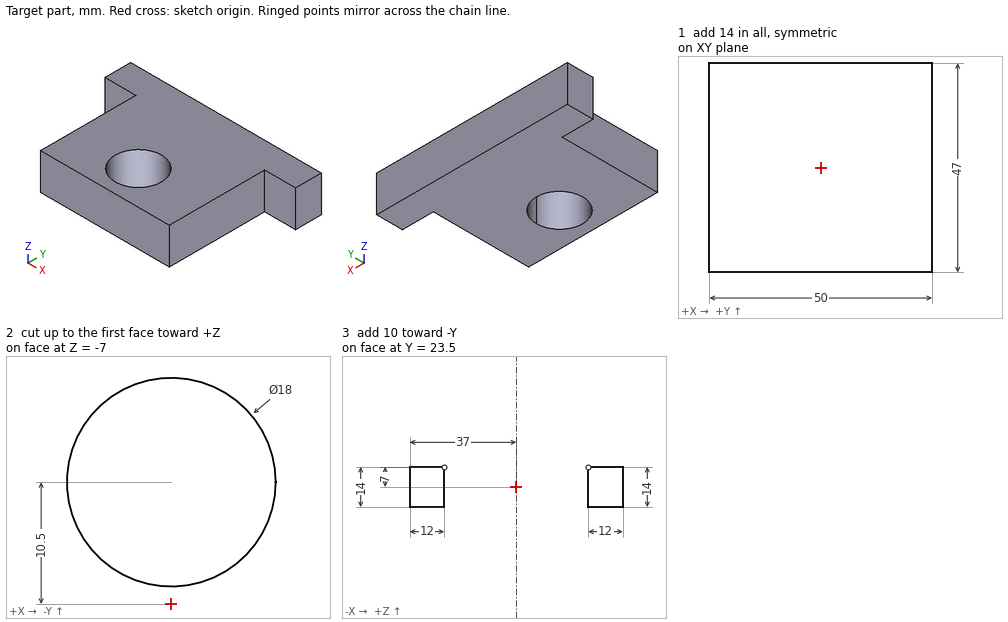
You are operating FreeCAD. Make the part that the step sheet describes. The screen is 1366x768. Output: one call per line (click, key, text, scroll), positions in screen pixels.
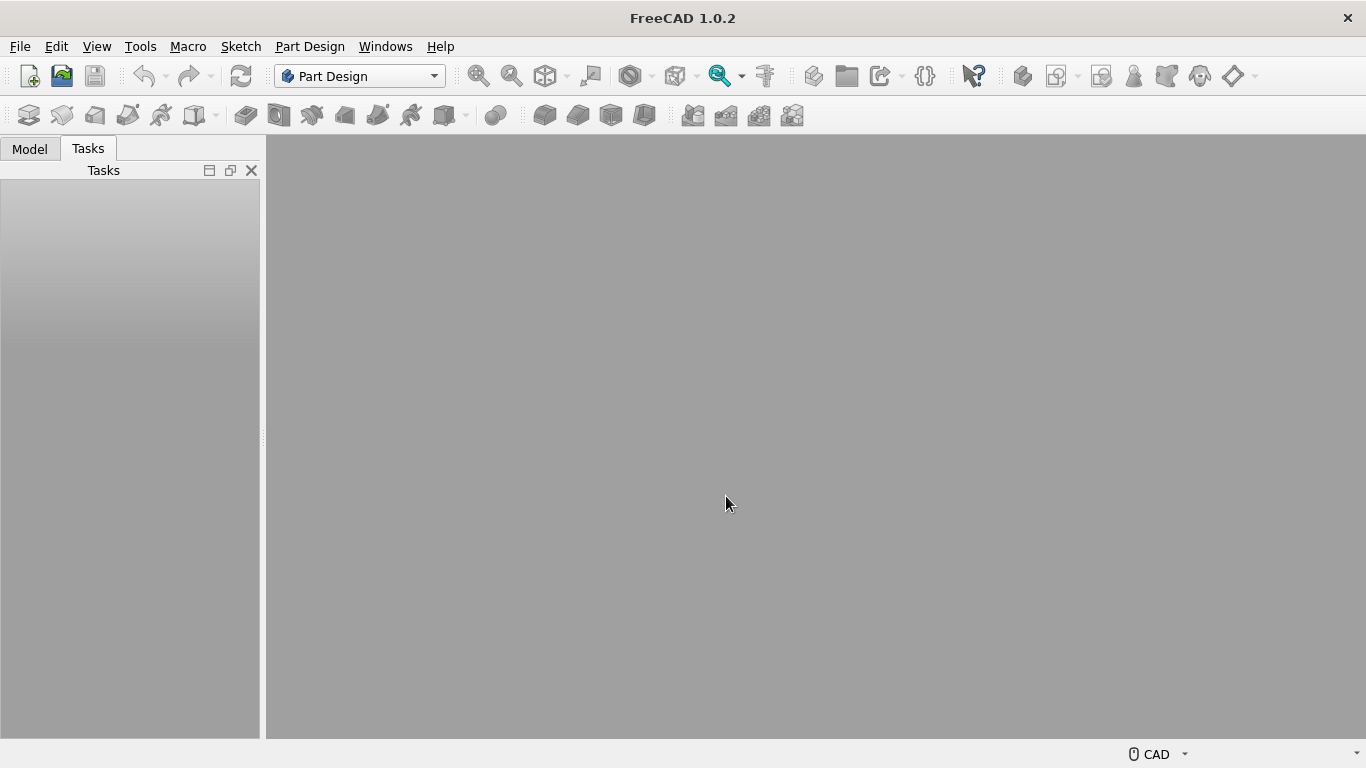
click(29, 76)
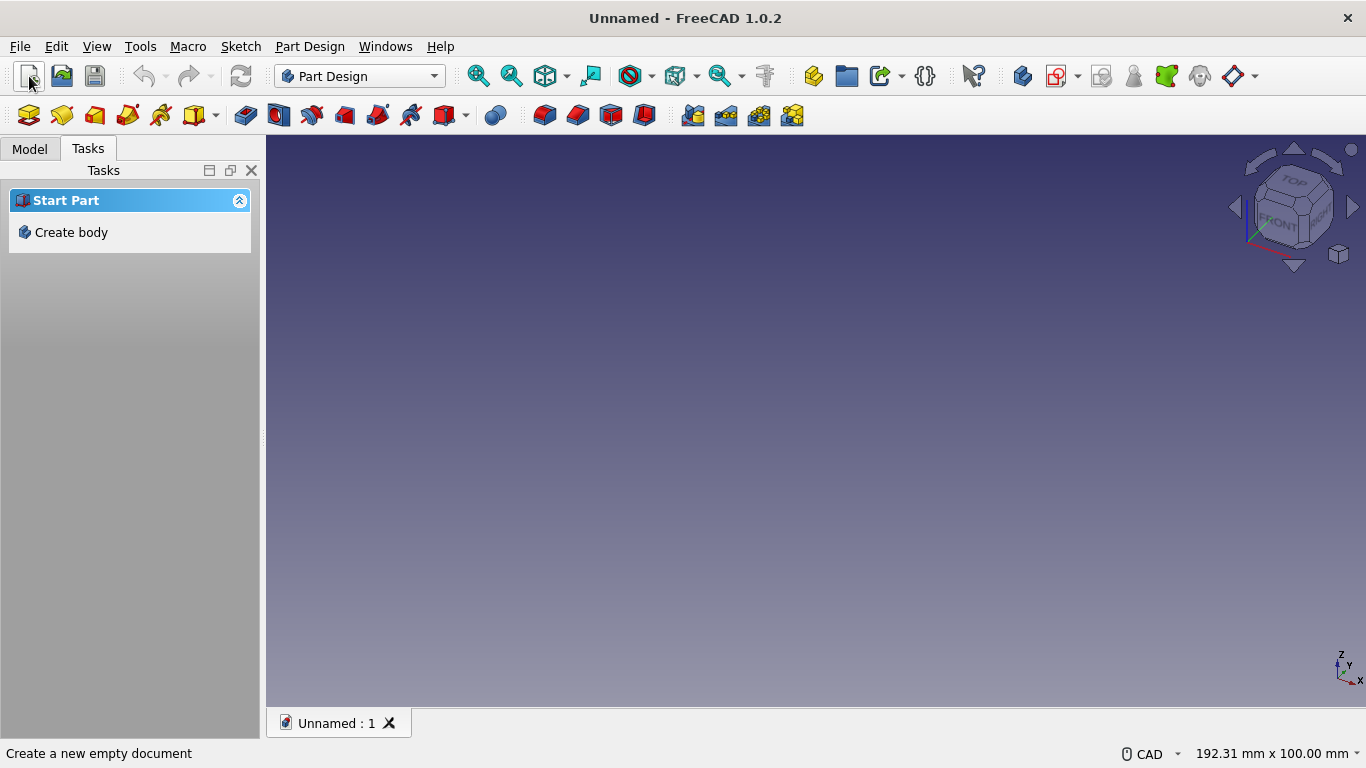
click(1056, 76)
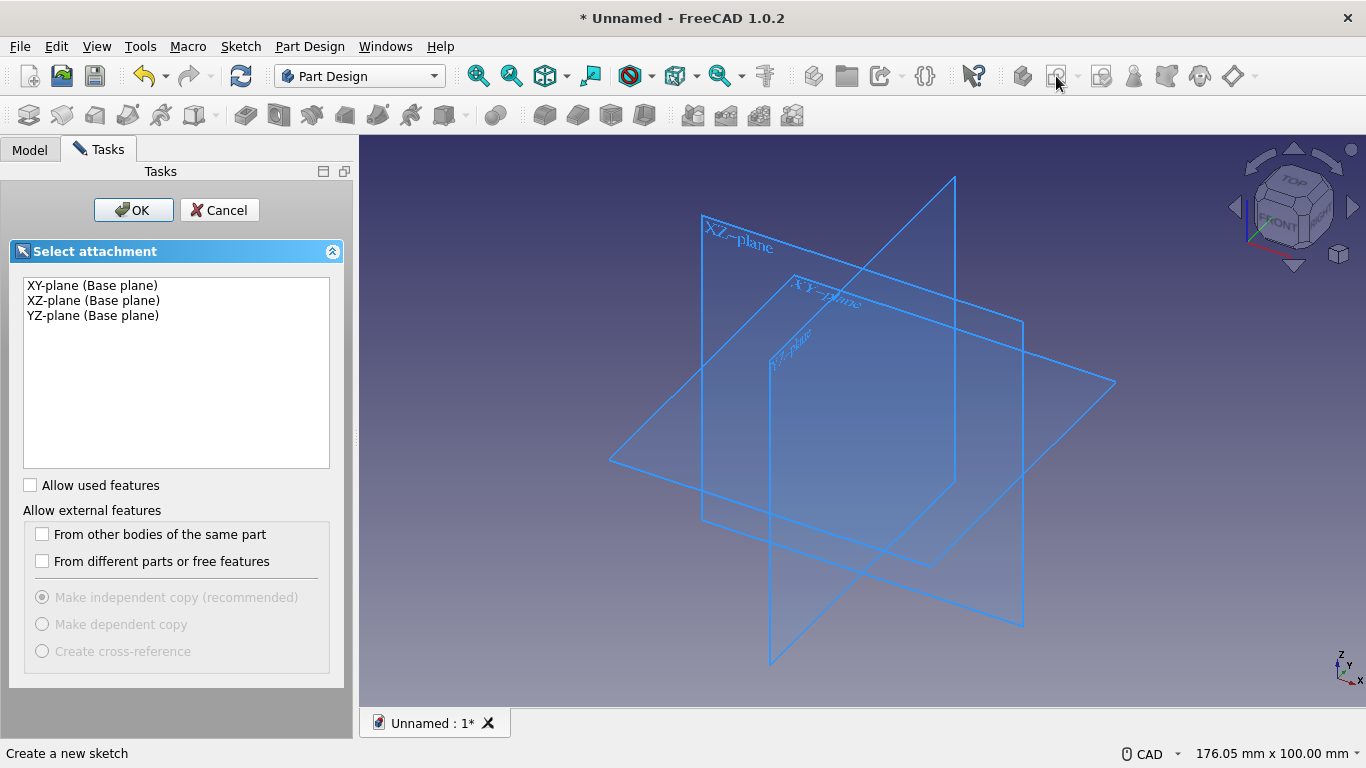
click(84, 286)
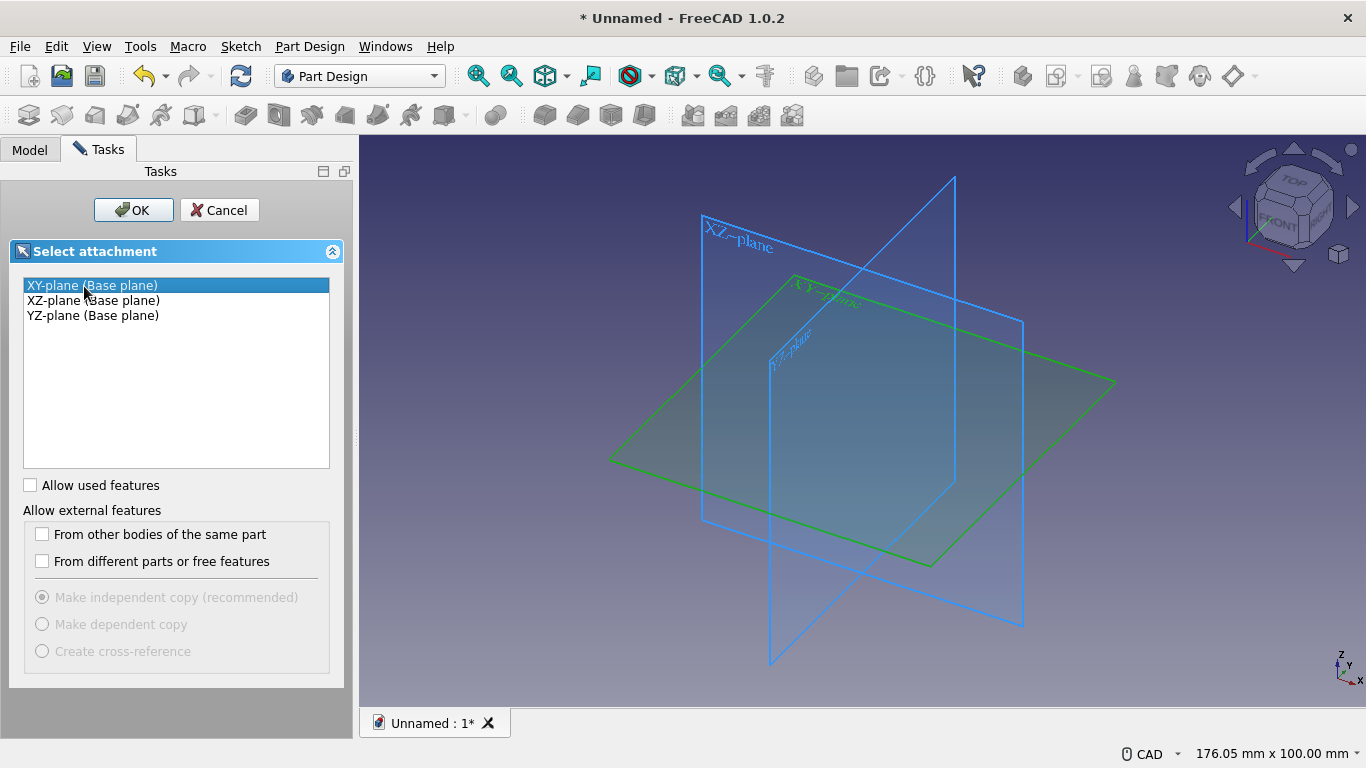
click(134, 210)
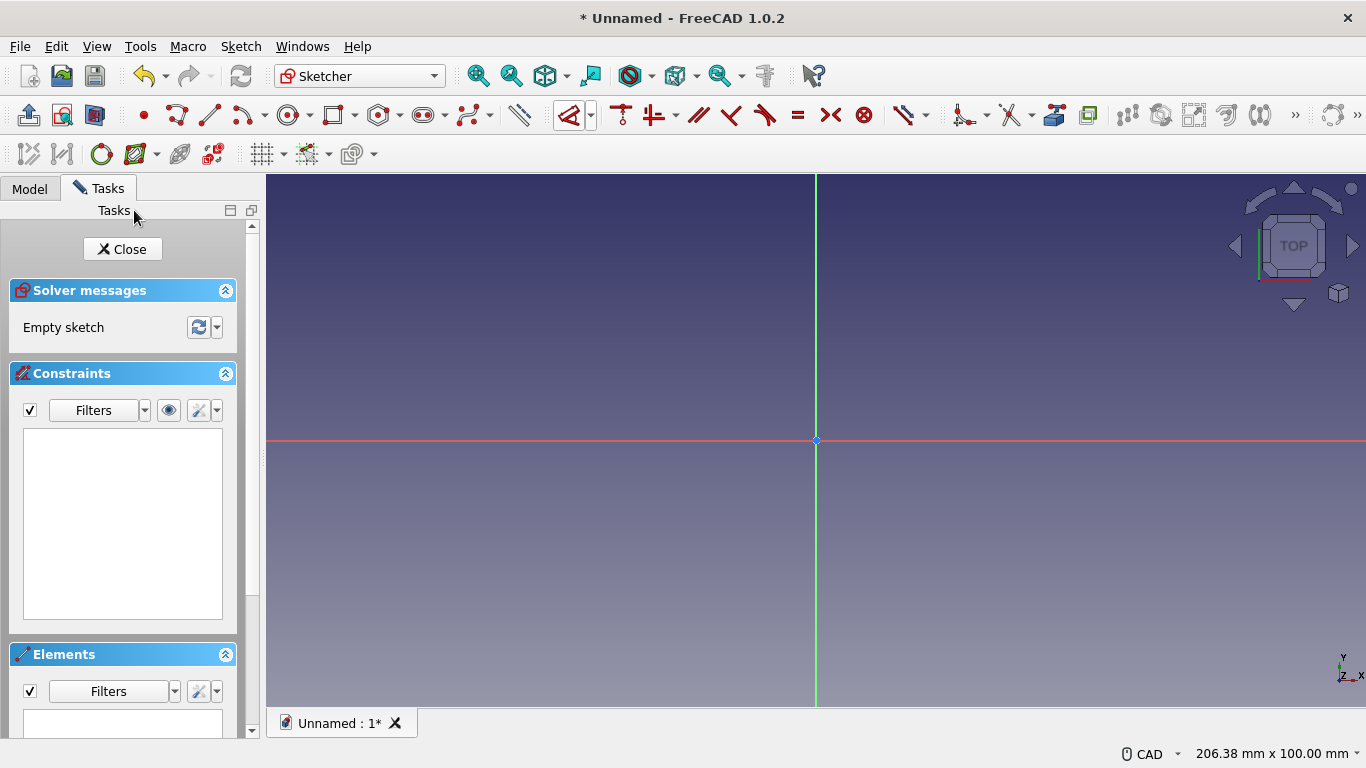
click(354, 116)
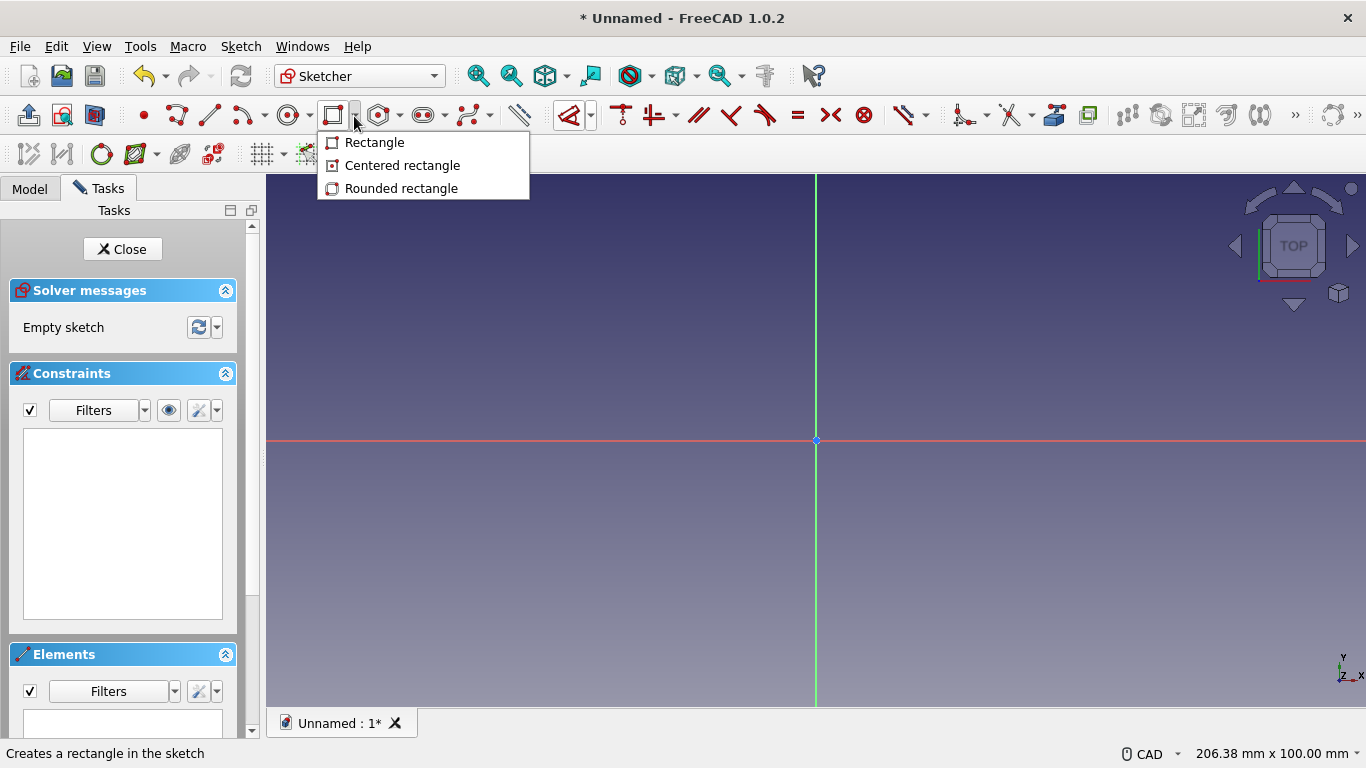
click(424, 166)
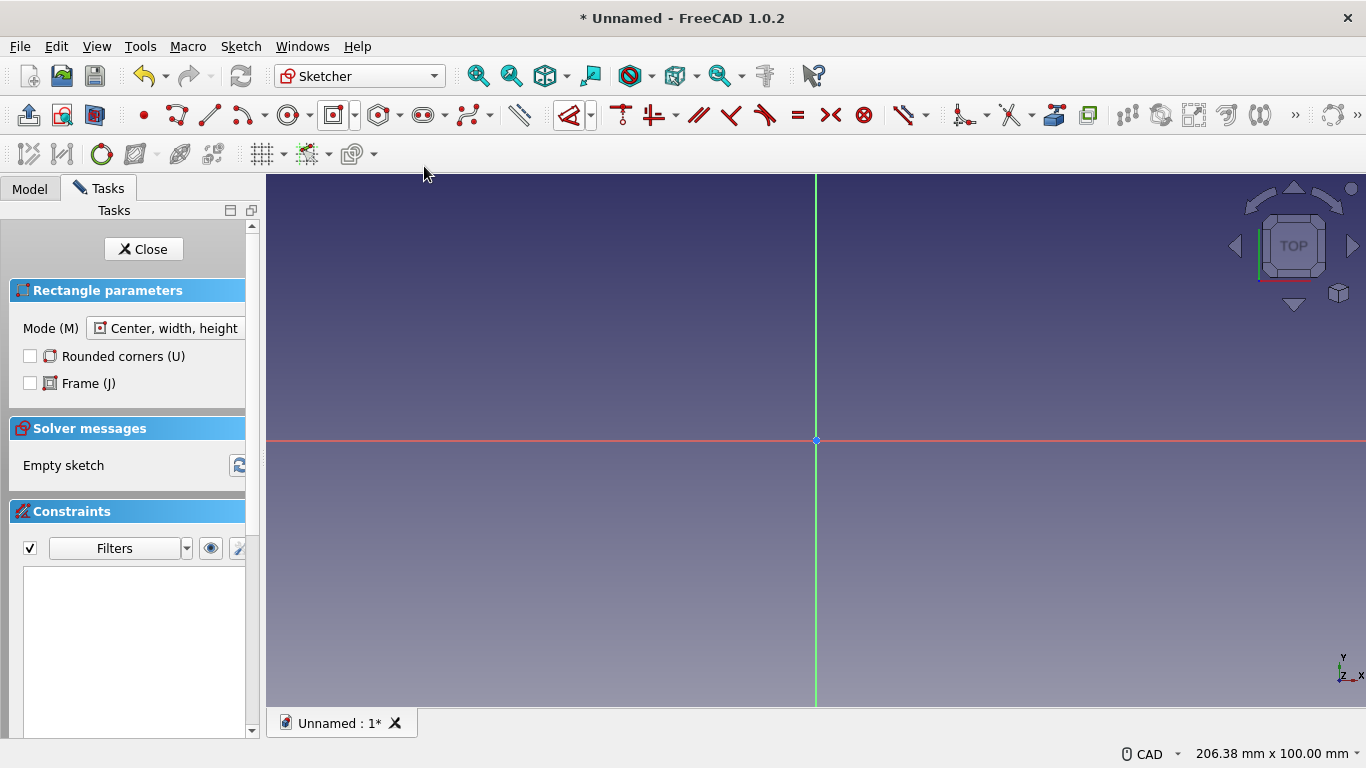
click(816, 440)
move(949, 315)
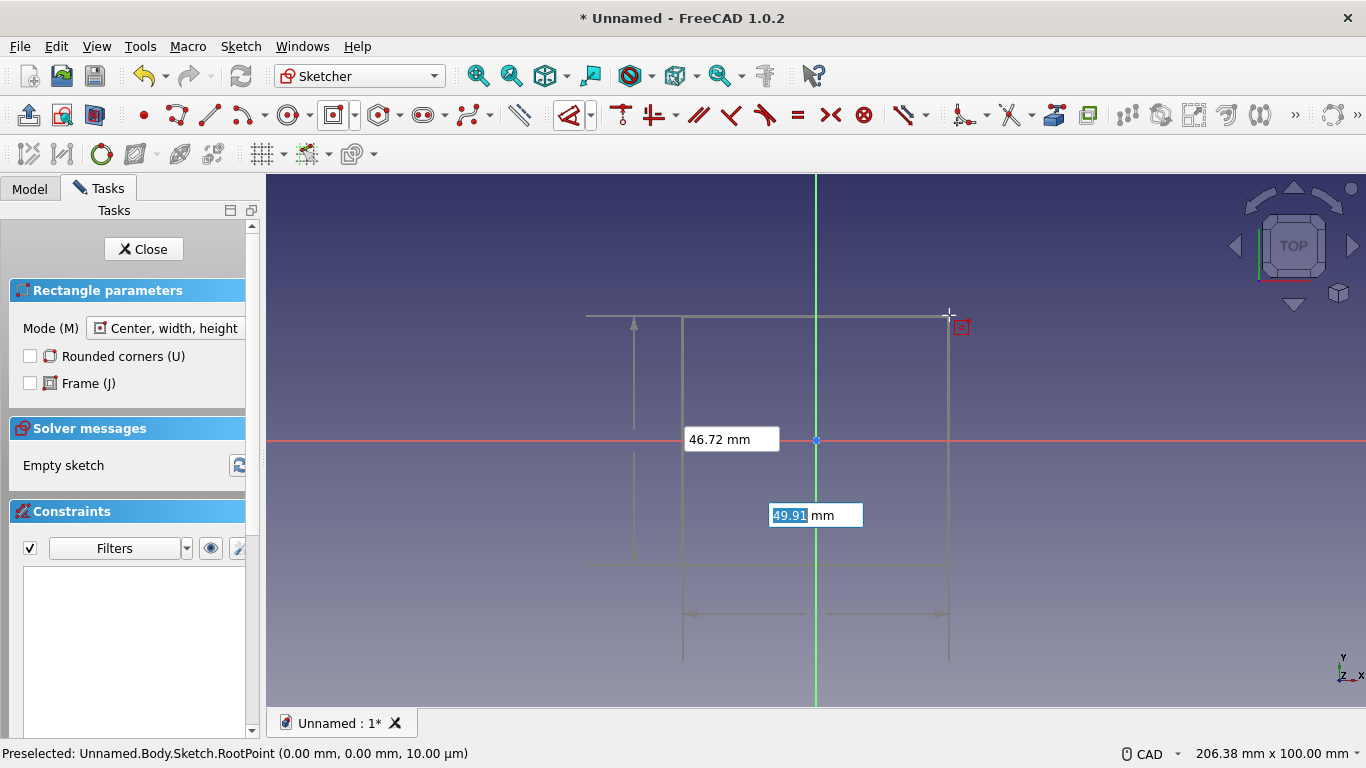
text(50)
key(Tab)
text(47)
key(Return)
key(Escape)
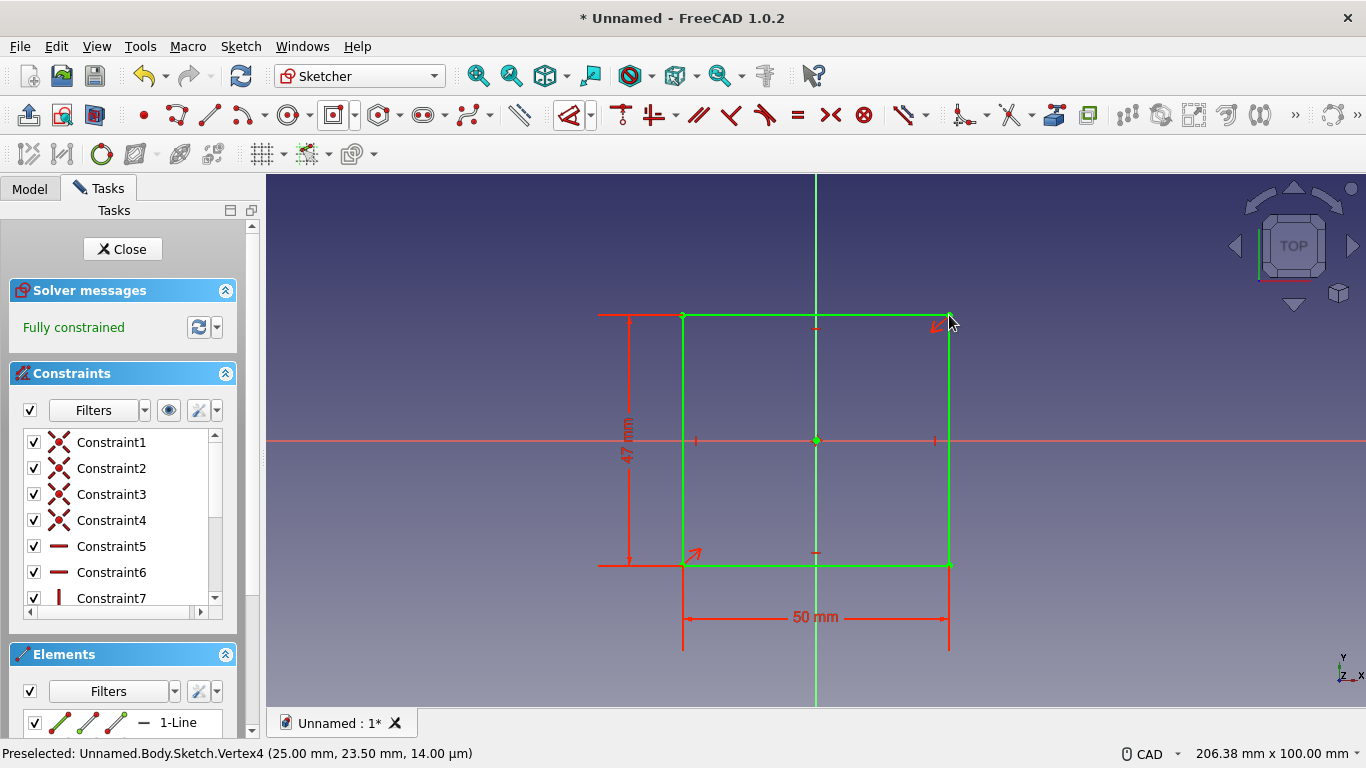
click(123, 249)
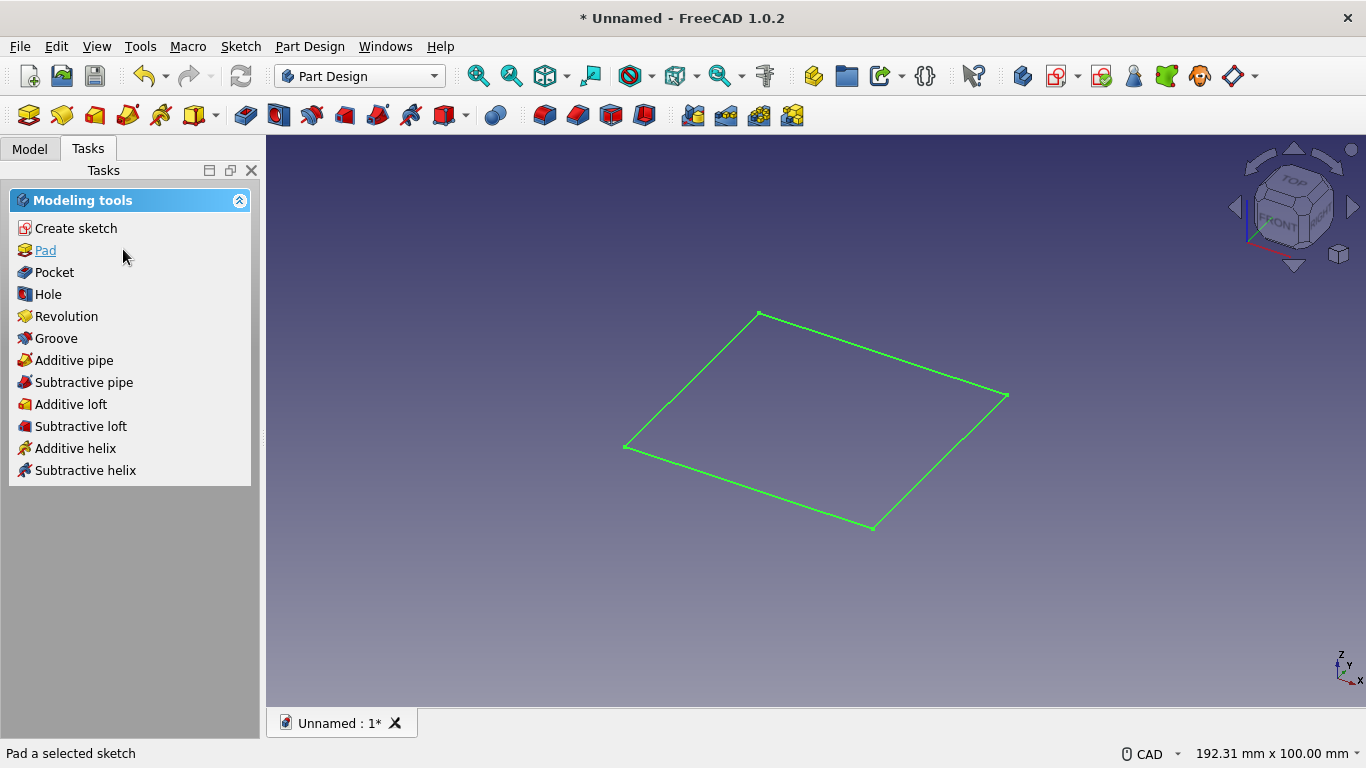
click(29, 116)